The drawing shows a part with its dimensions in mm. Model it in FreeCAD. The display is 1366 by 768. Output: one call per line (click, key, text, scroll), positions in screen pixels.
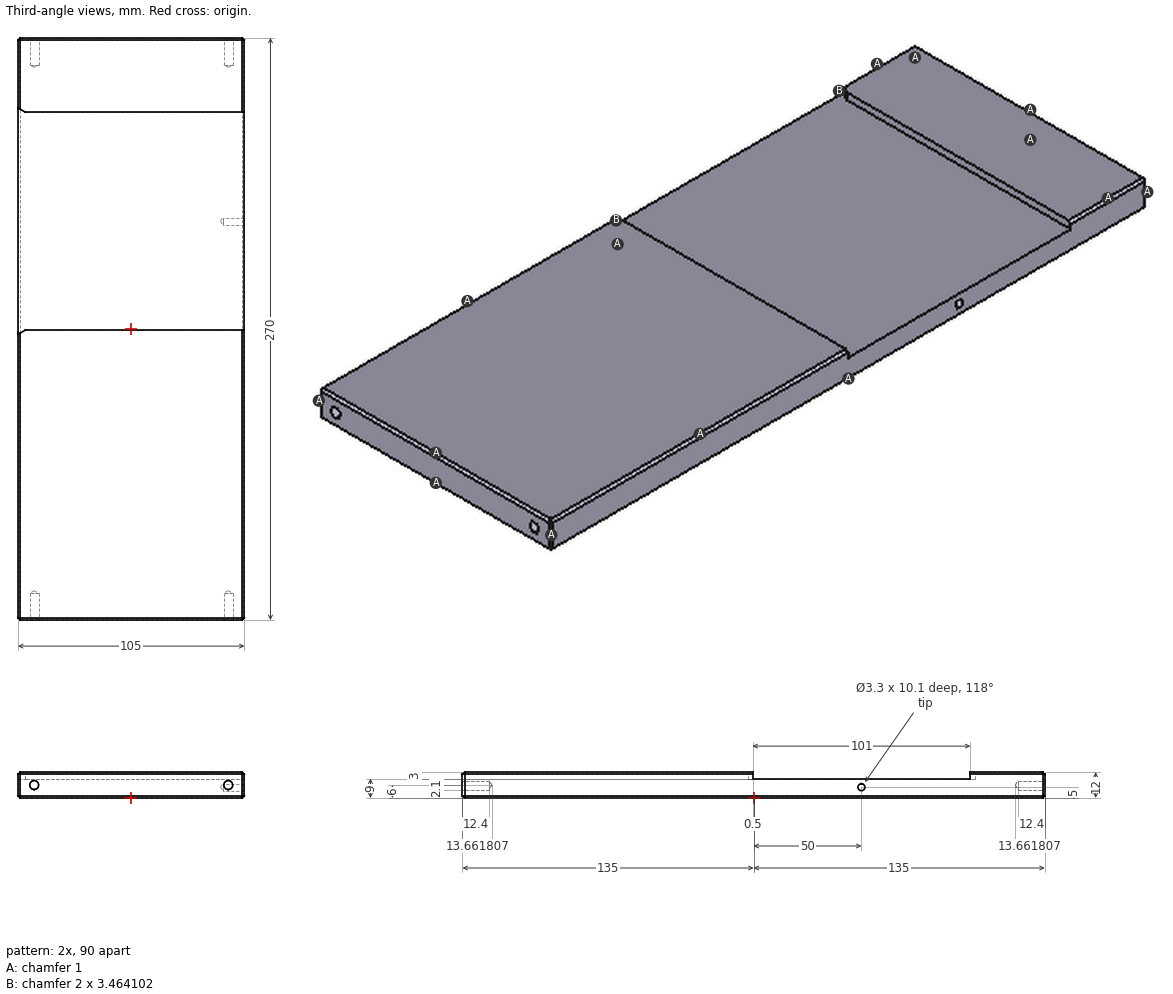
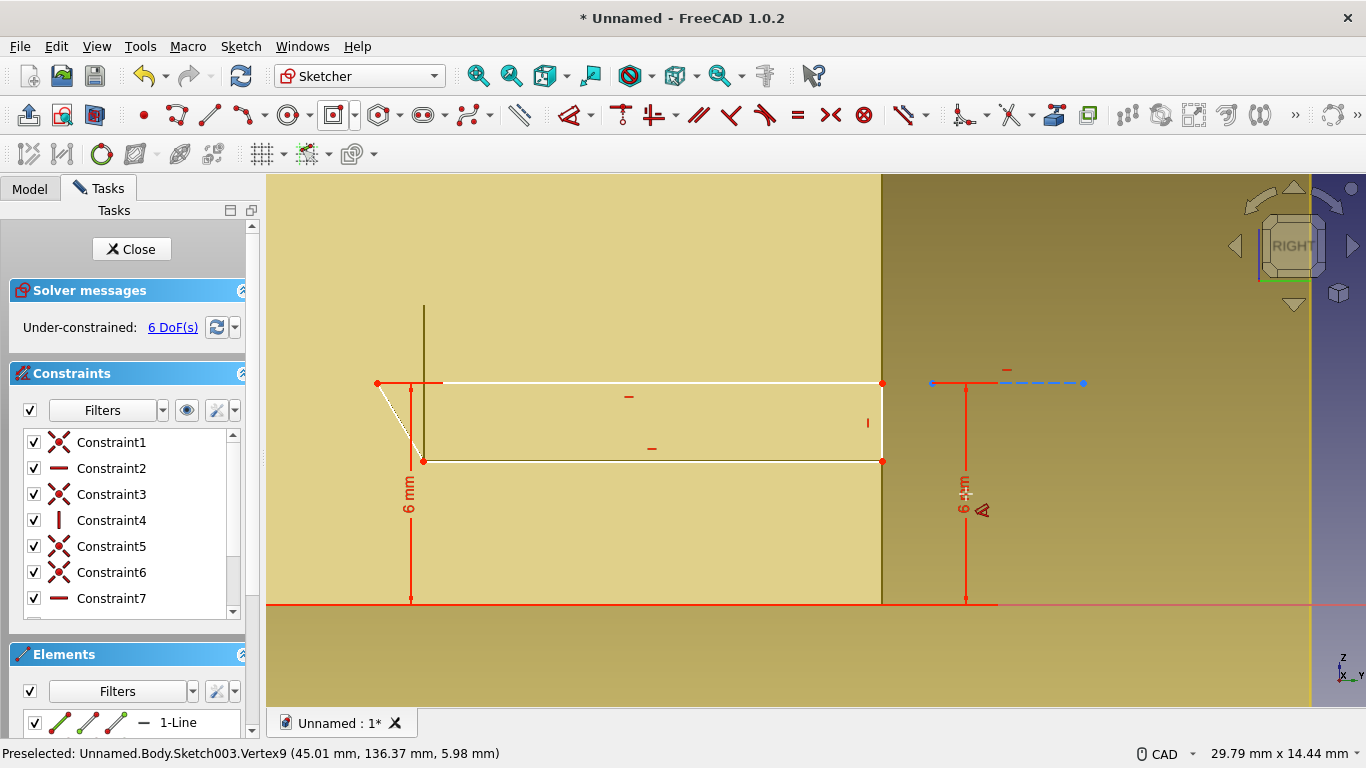
click(882, 438)
click(916, 423)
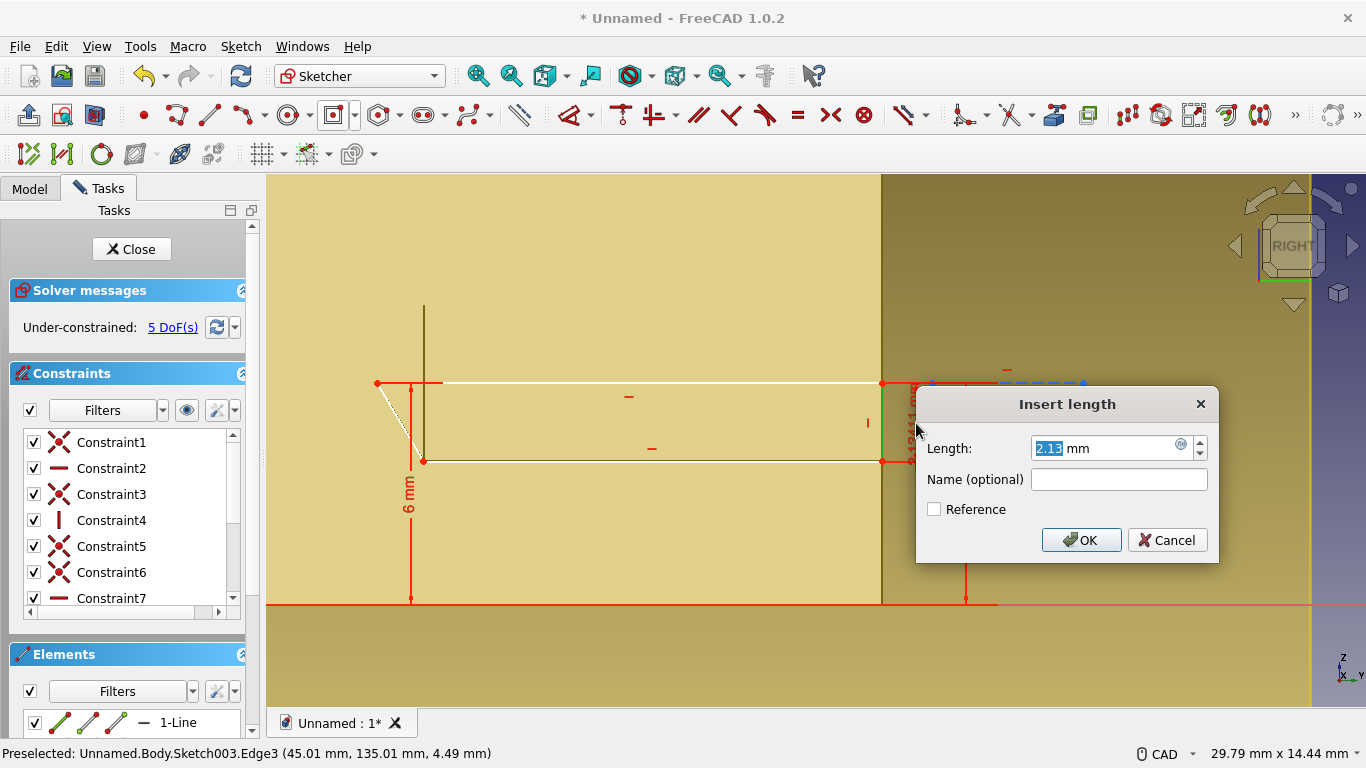
text(2.1)
key(Return)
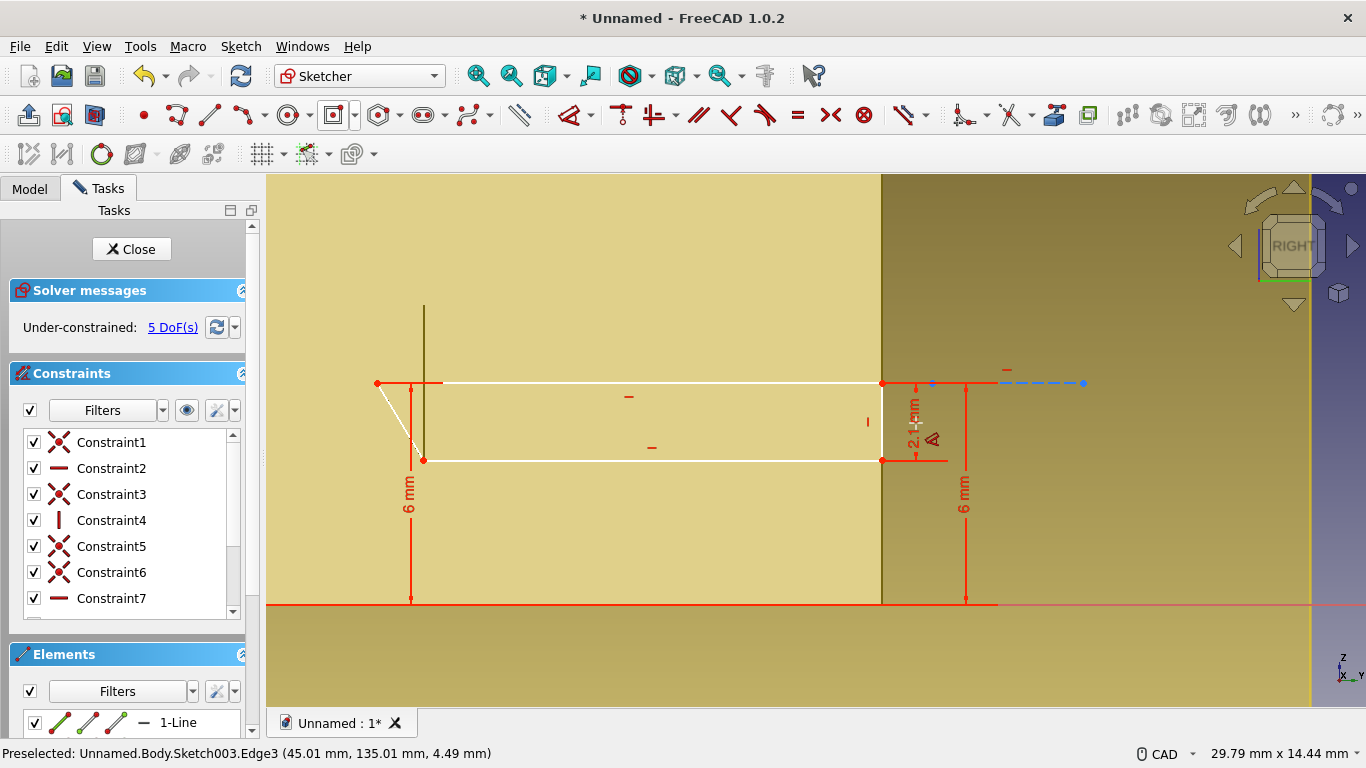
click(561, 461)
click(653, 495)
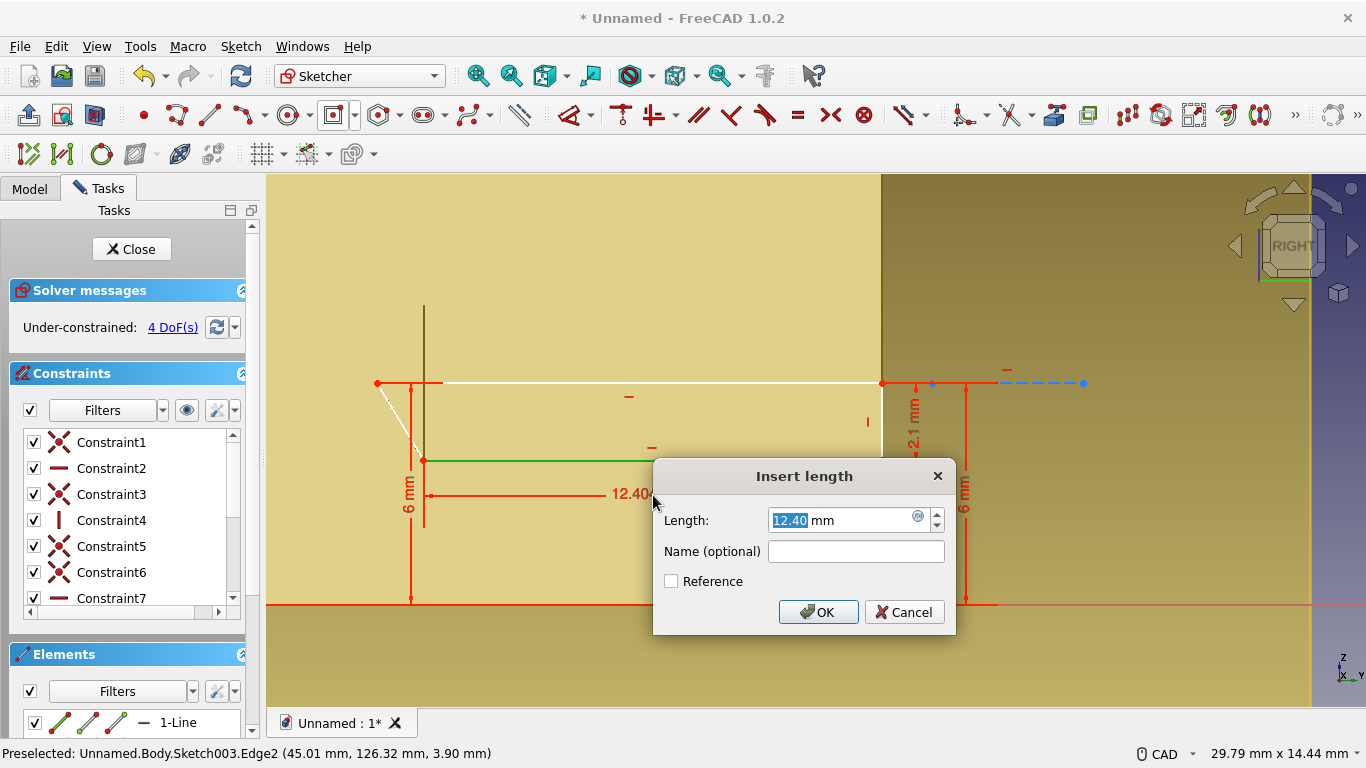
text(12.4)
key(Return)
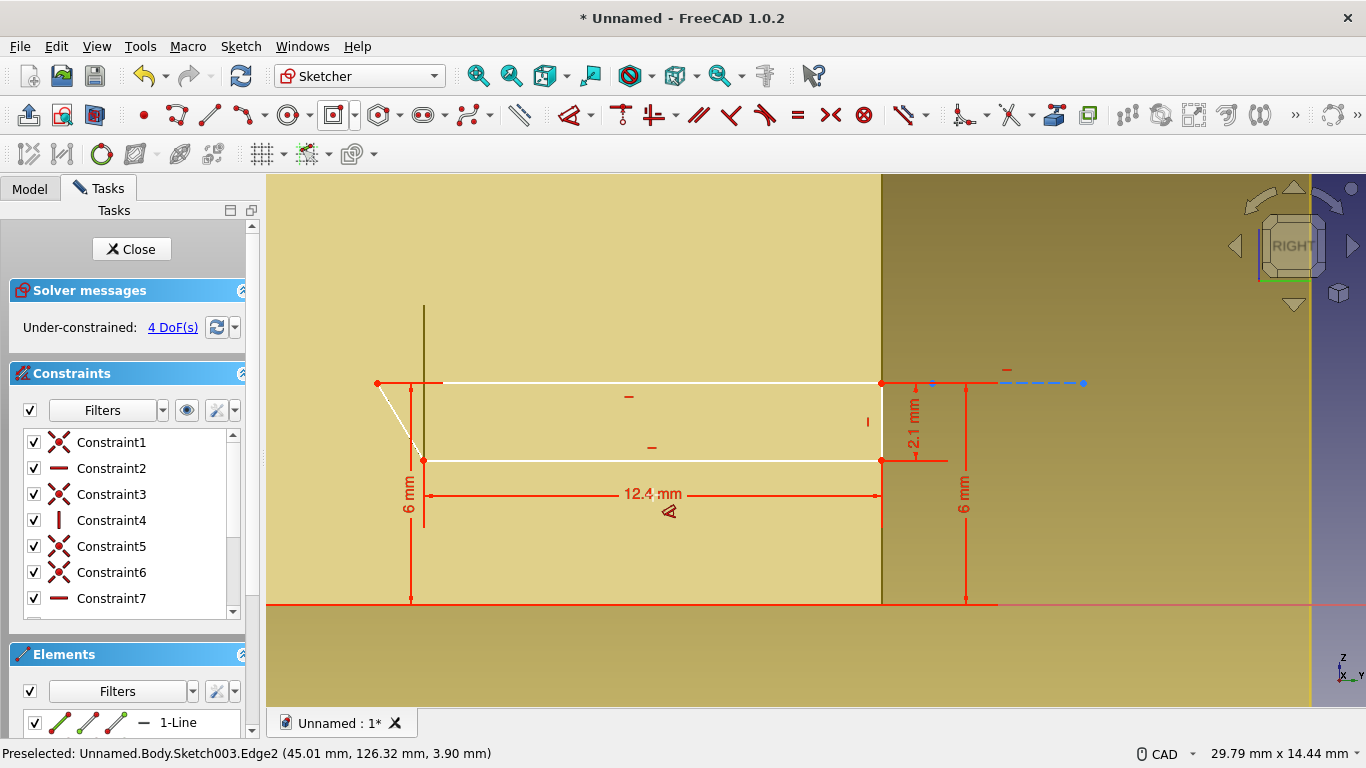
click(882, 461)
click(588, 639)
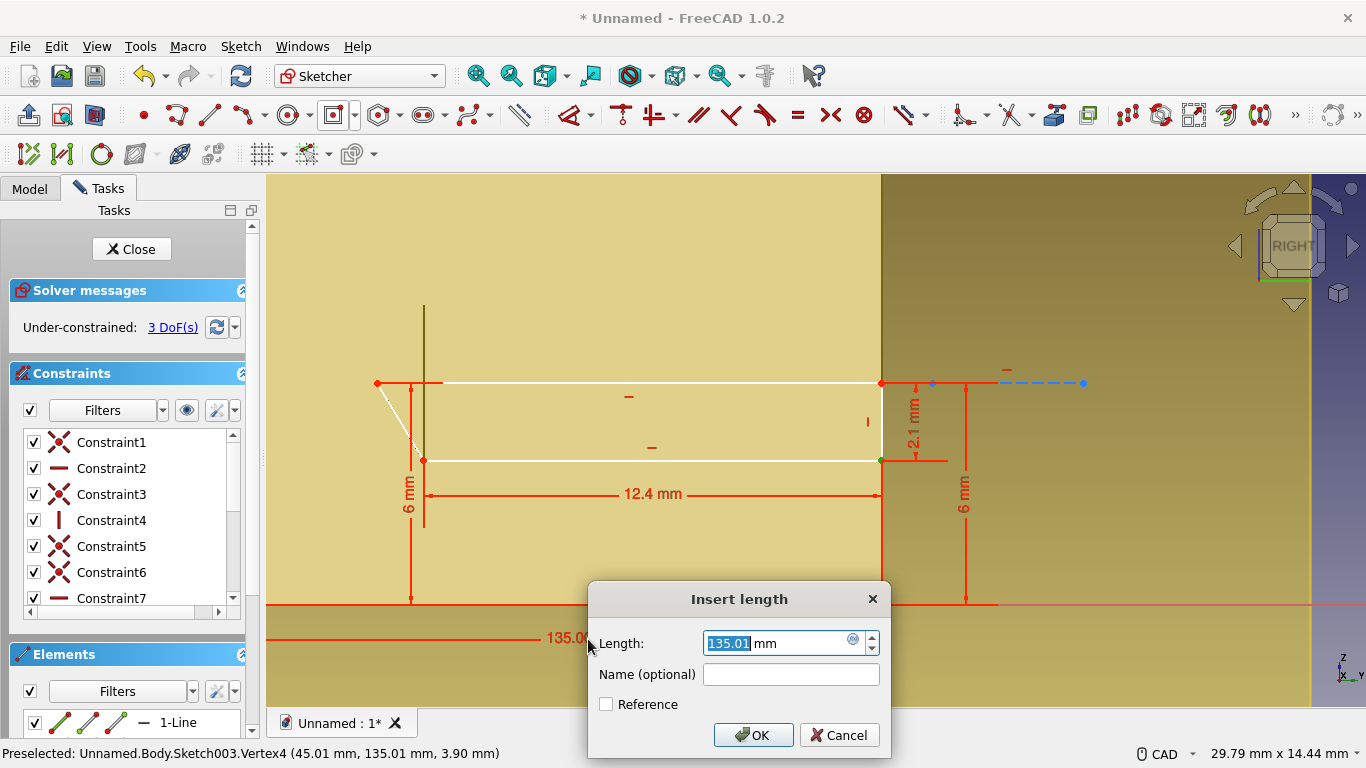
text(135)
key(Return)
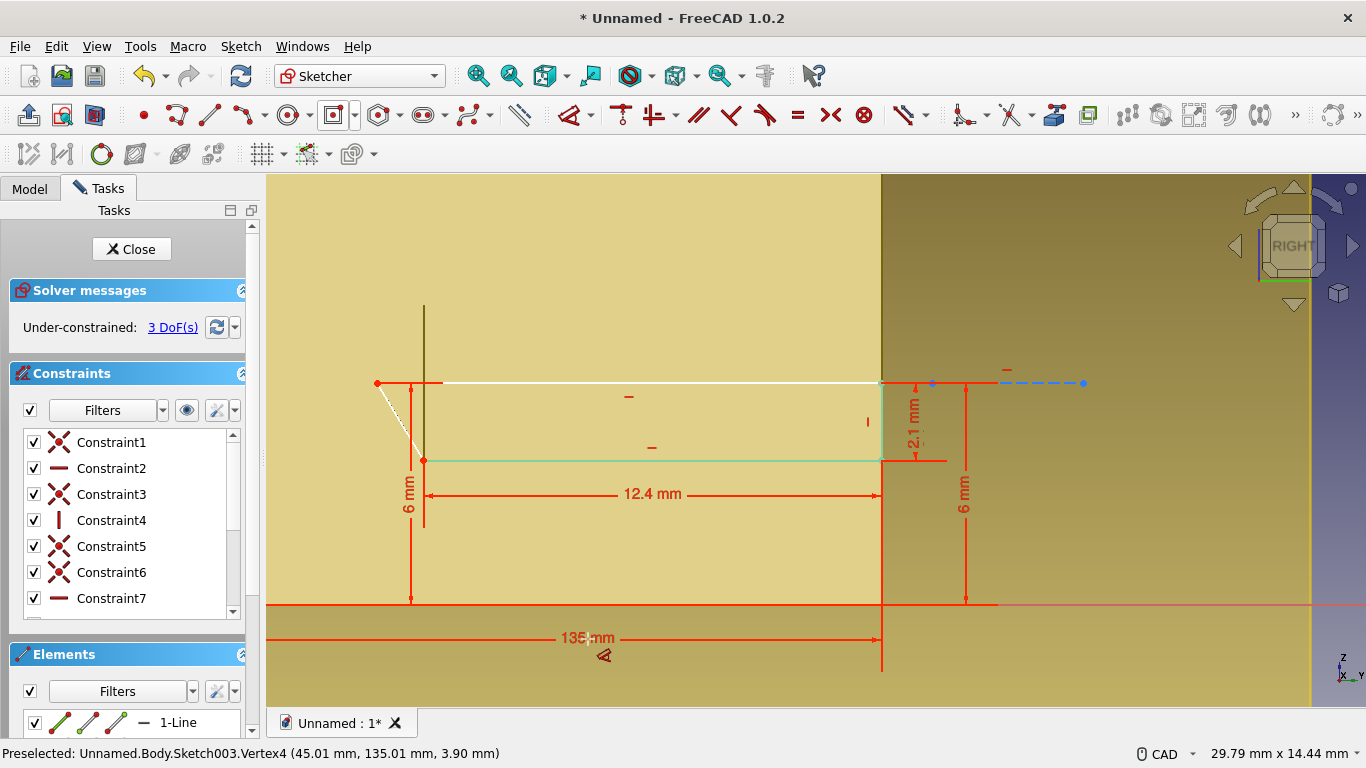
click(730, 383)
click(629, 349)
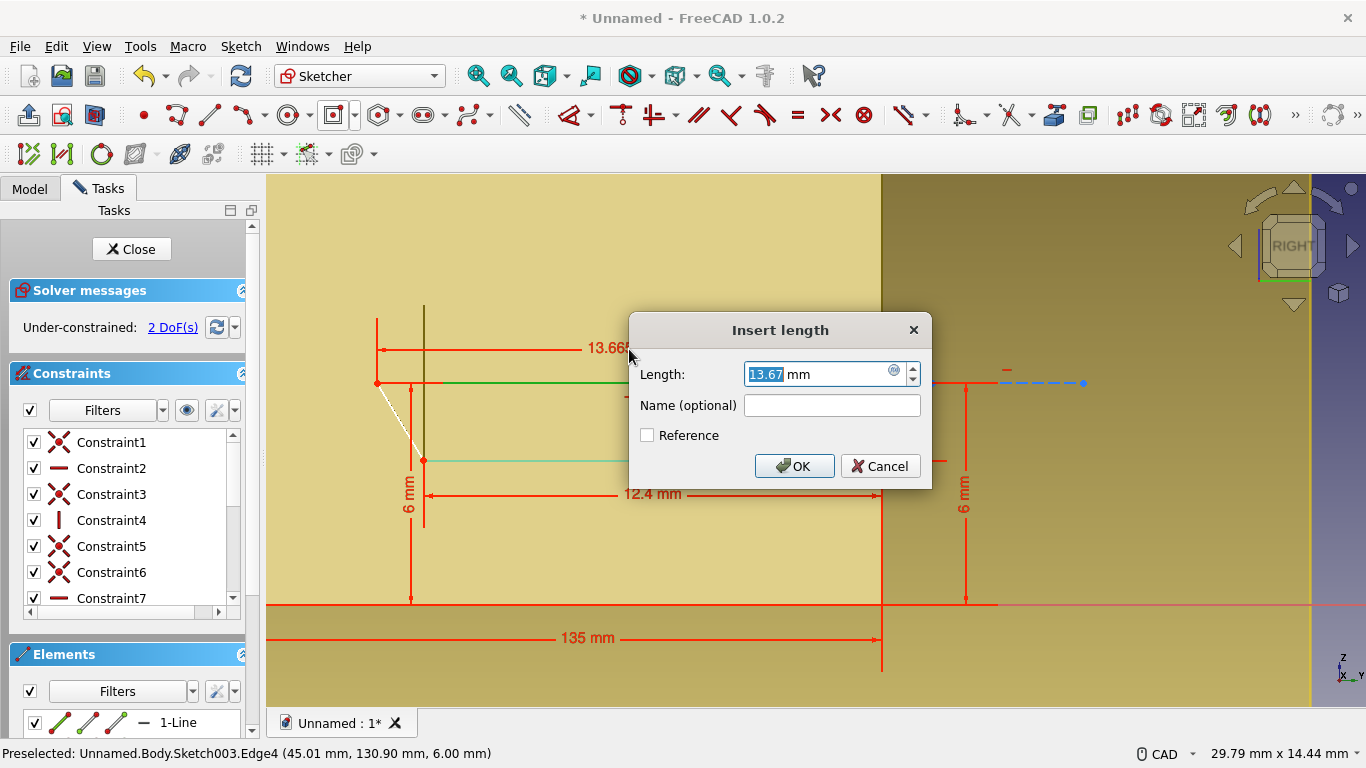
text(13.661807)
key(Return)
key(Escape)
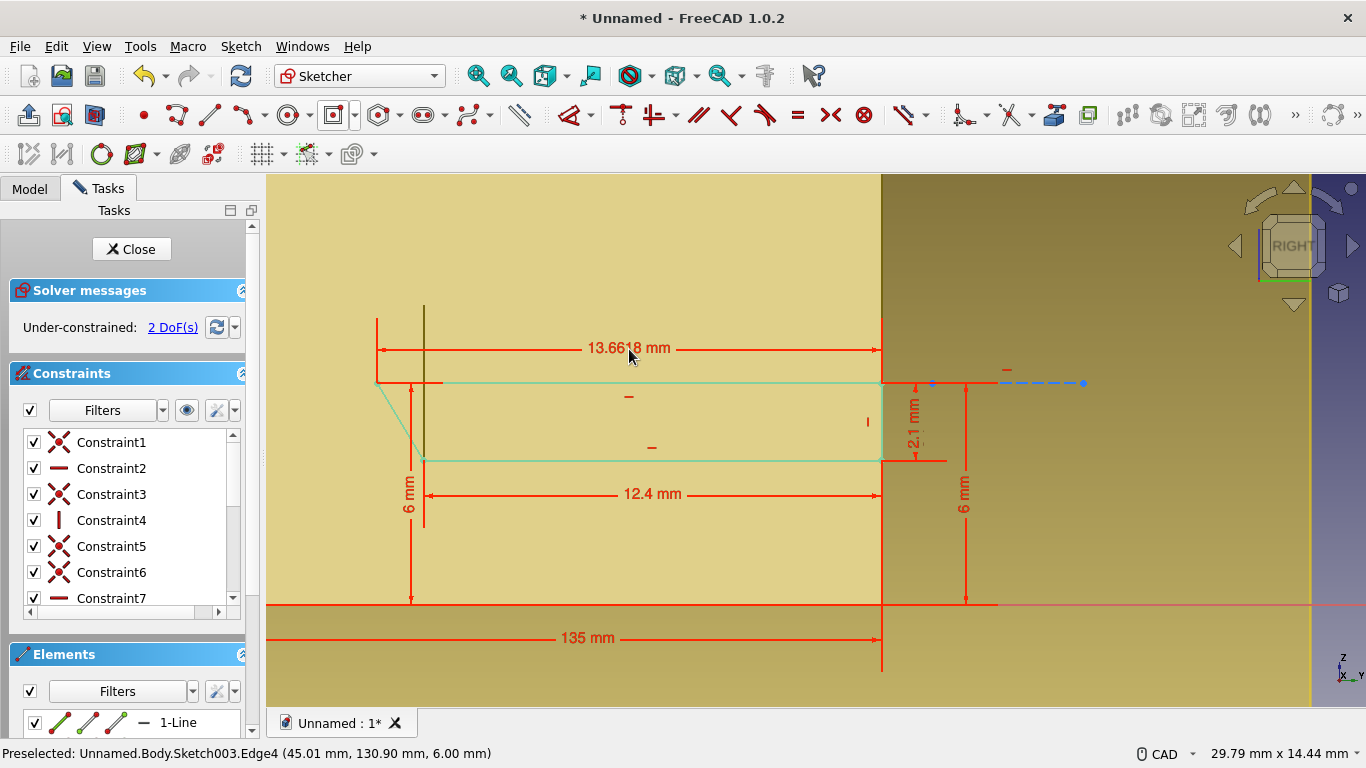
click(132, 249)